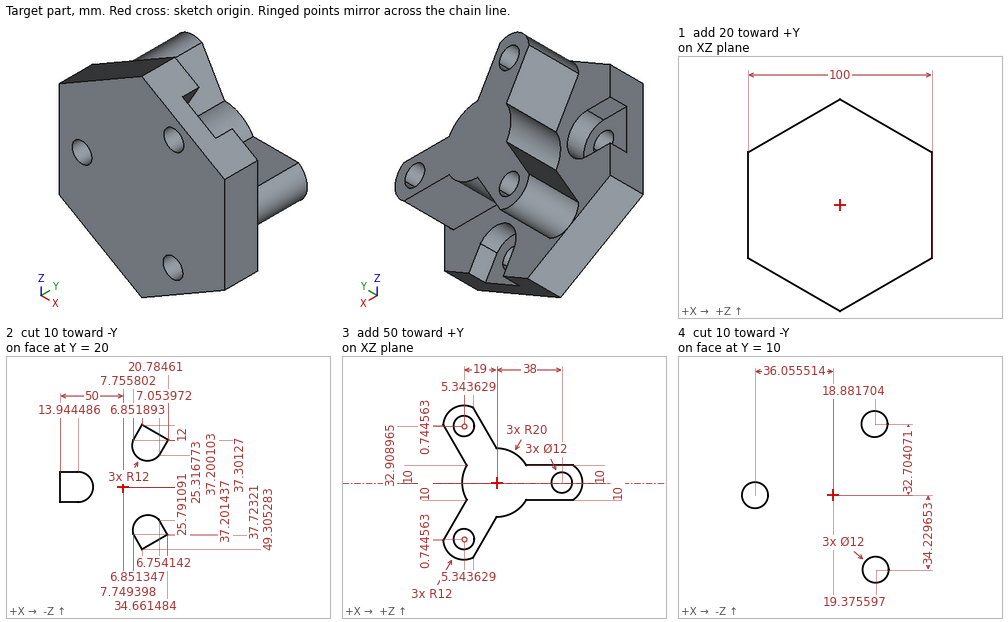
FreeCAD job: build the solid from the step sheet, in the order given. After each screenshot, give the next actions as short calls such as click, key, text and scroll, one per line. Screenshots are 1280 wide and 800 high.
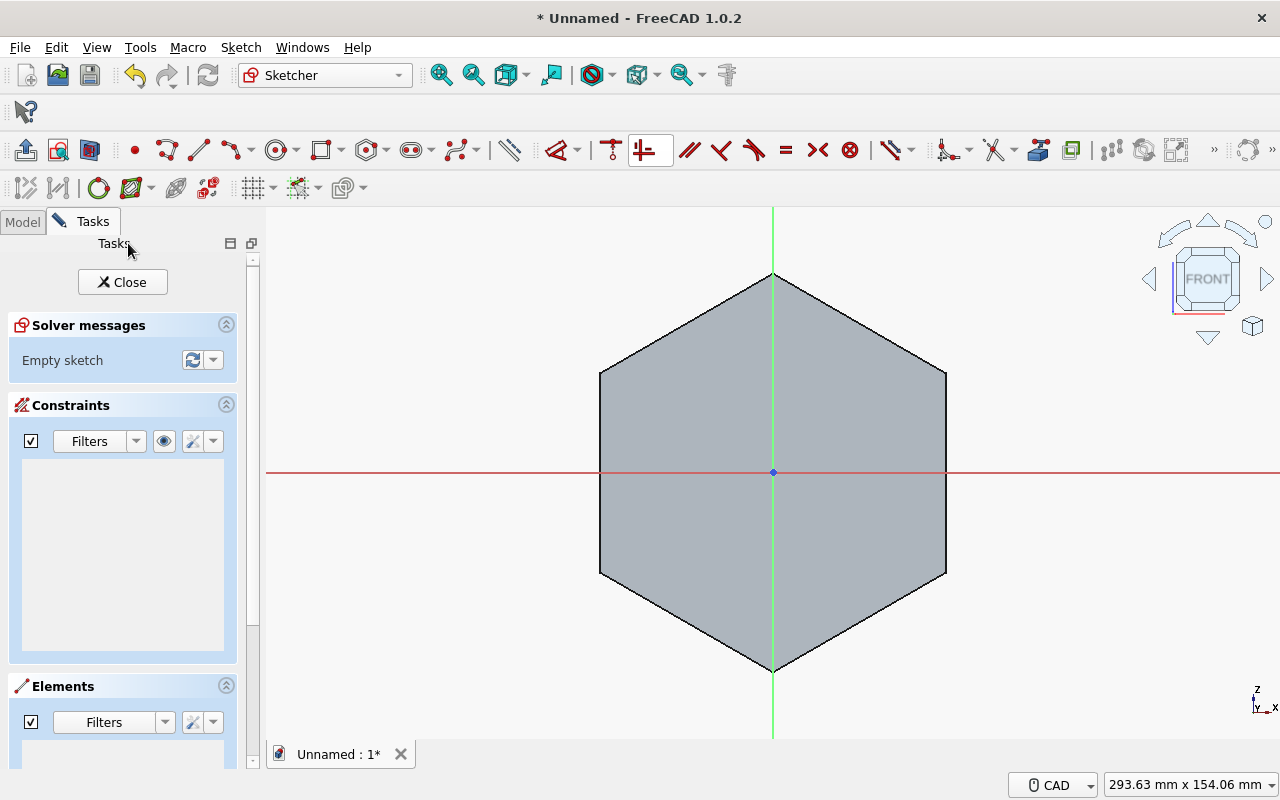
click(200, 150)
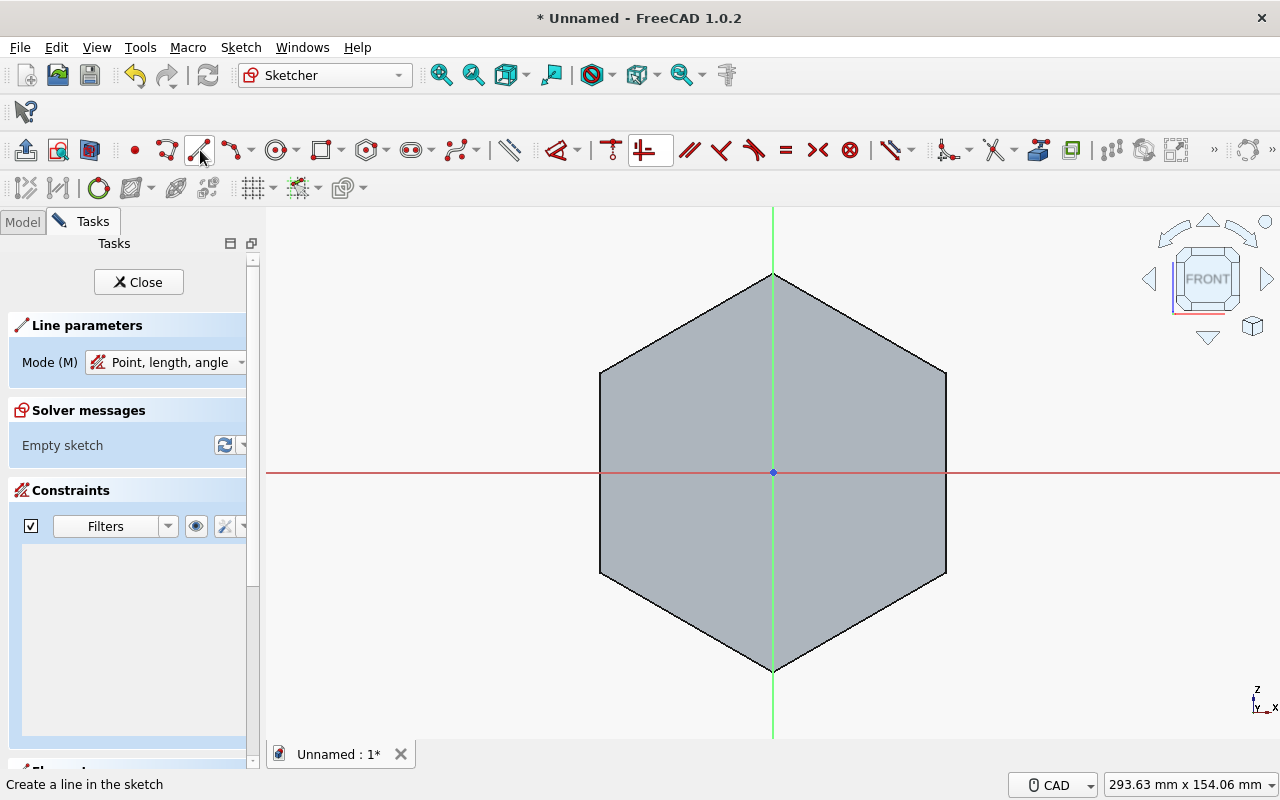
click(833, 438)
click(927, 438)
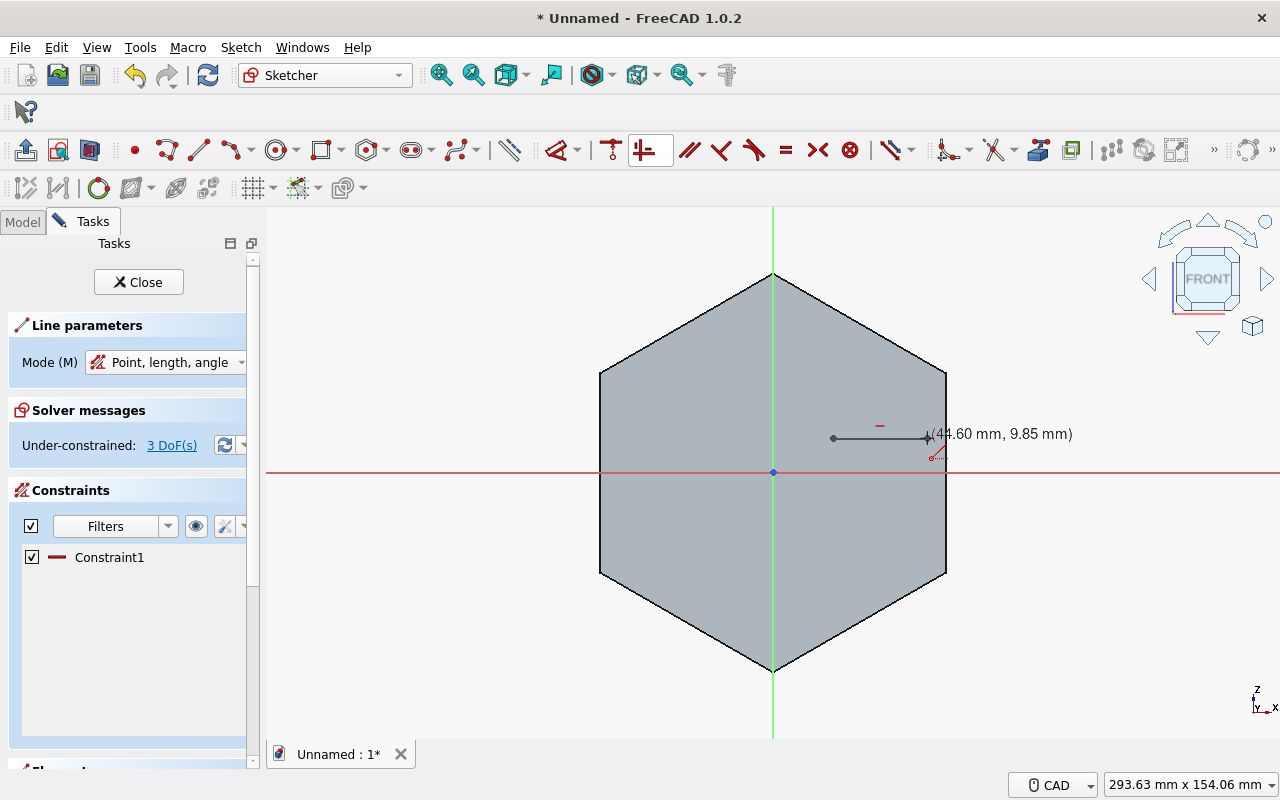
click(927, 508)
click(833, 508)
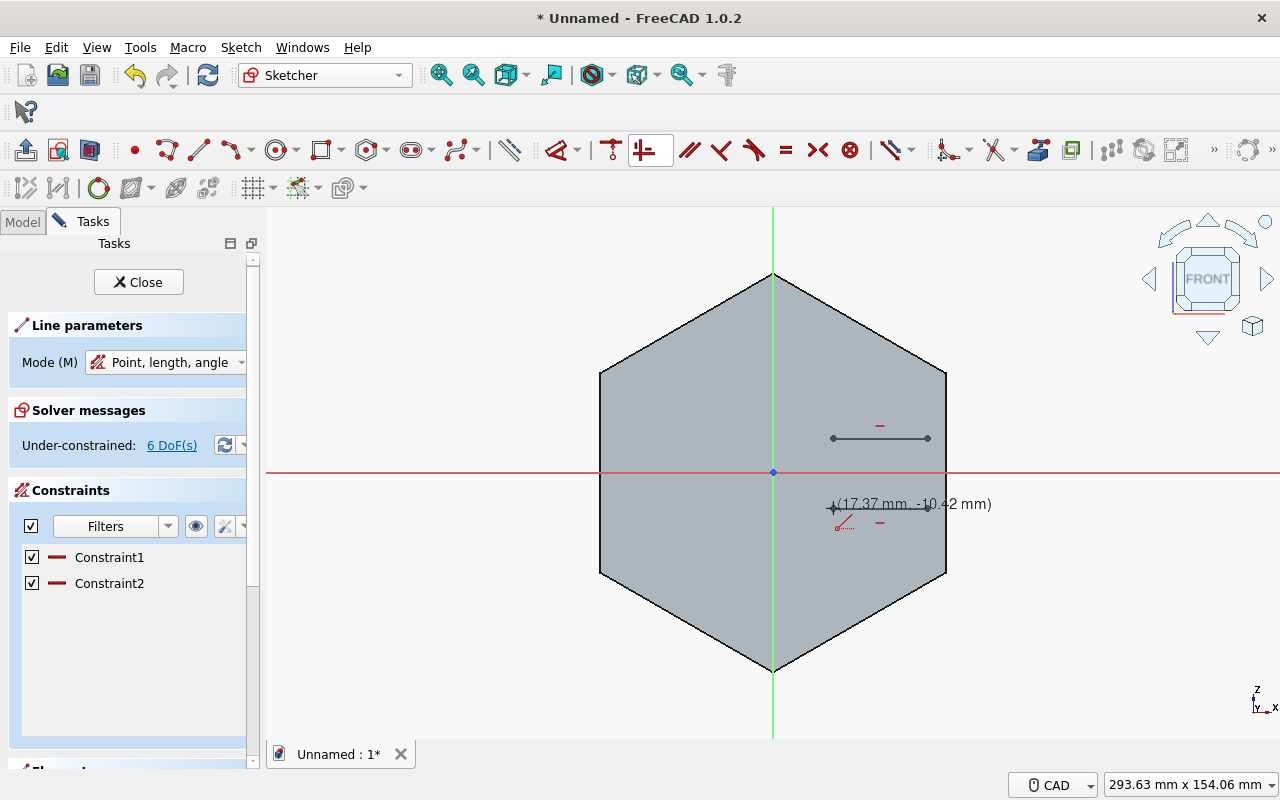
click(773, 542)
click(726, 624)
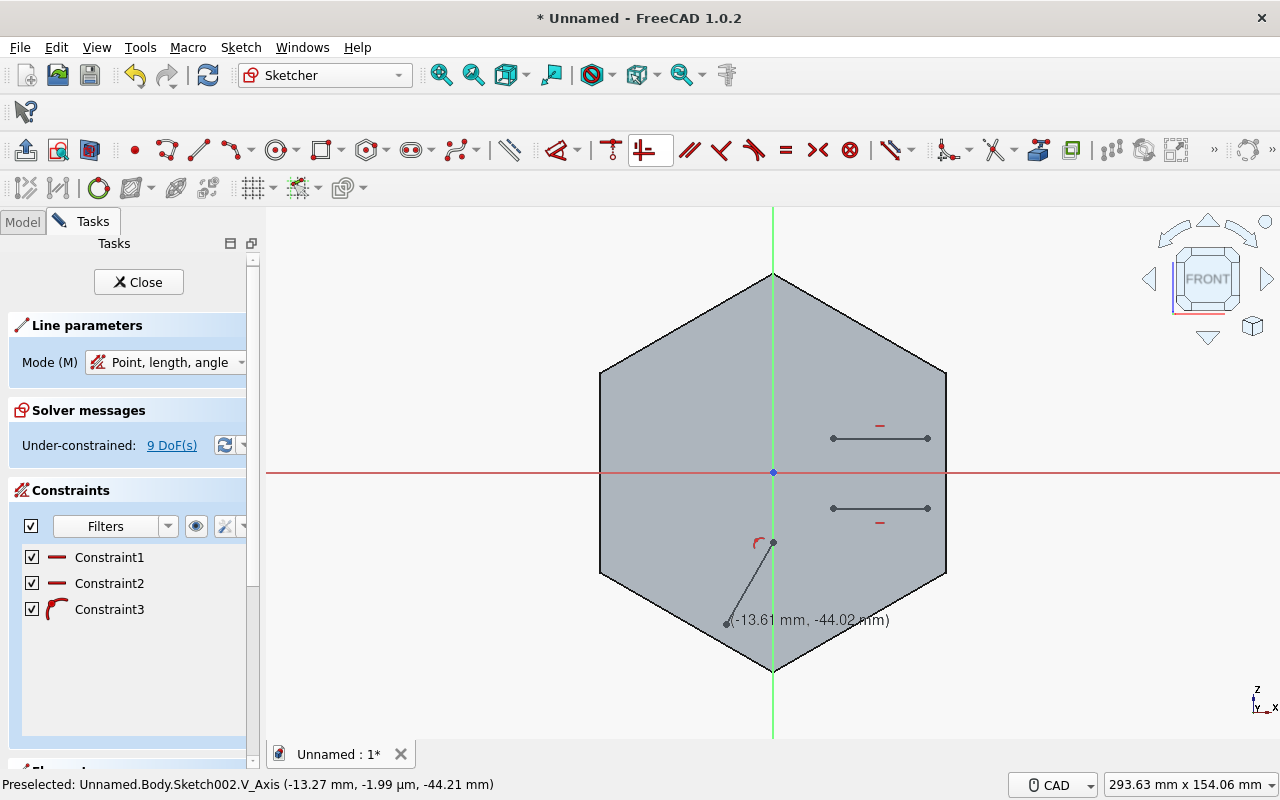
click(666, 589)
click(713, 508)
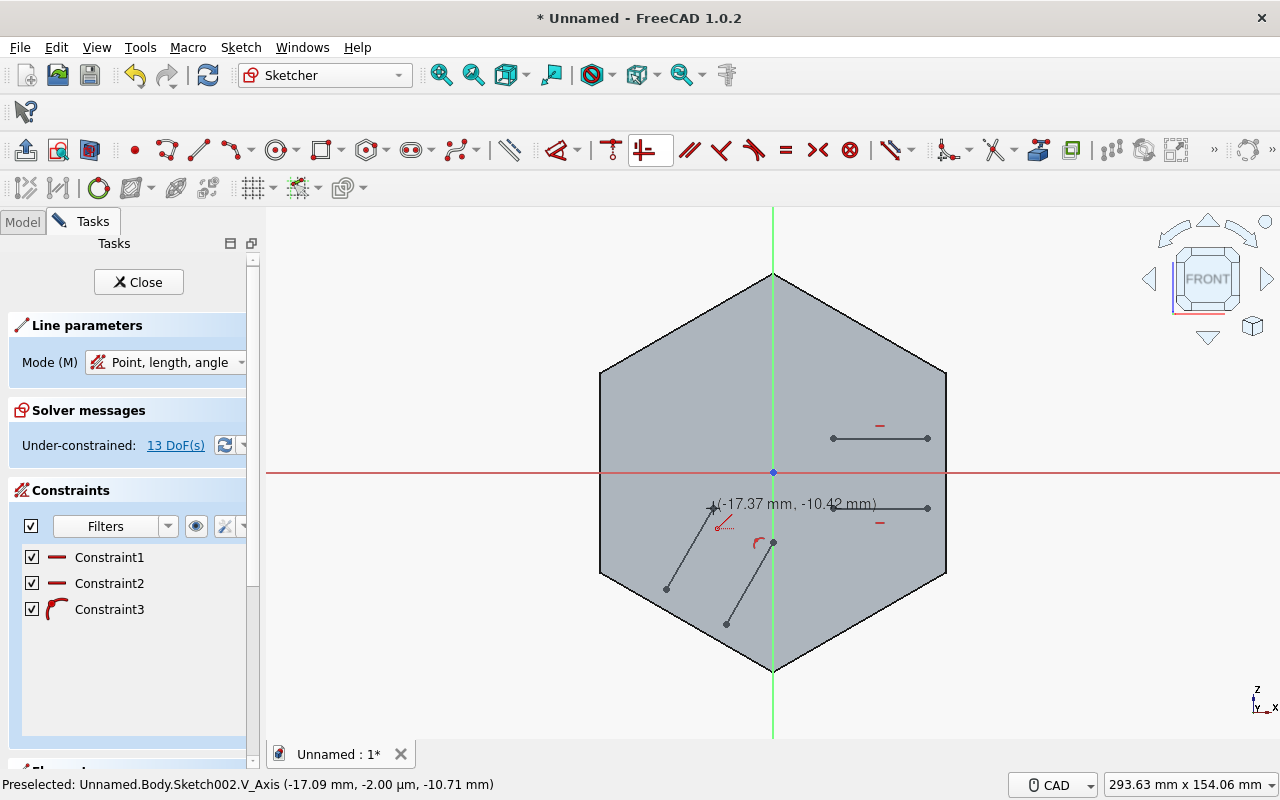
click(713, 438)
click(666, 357)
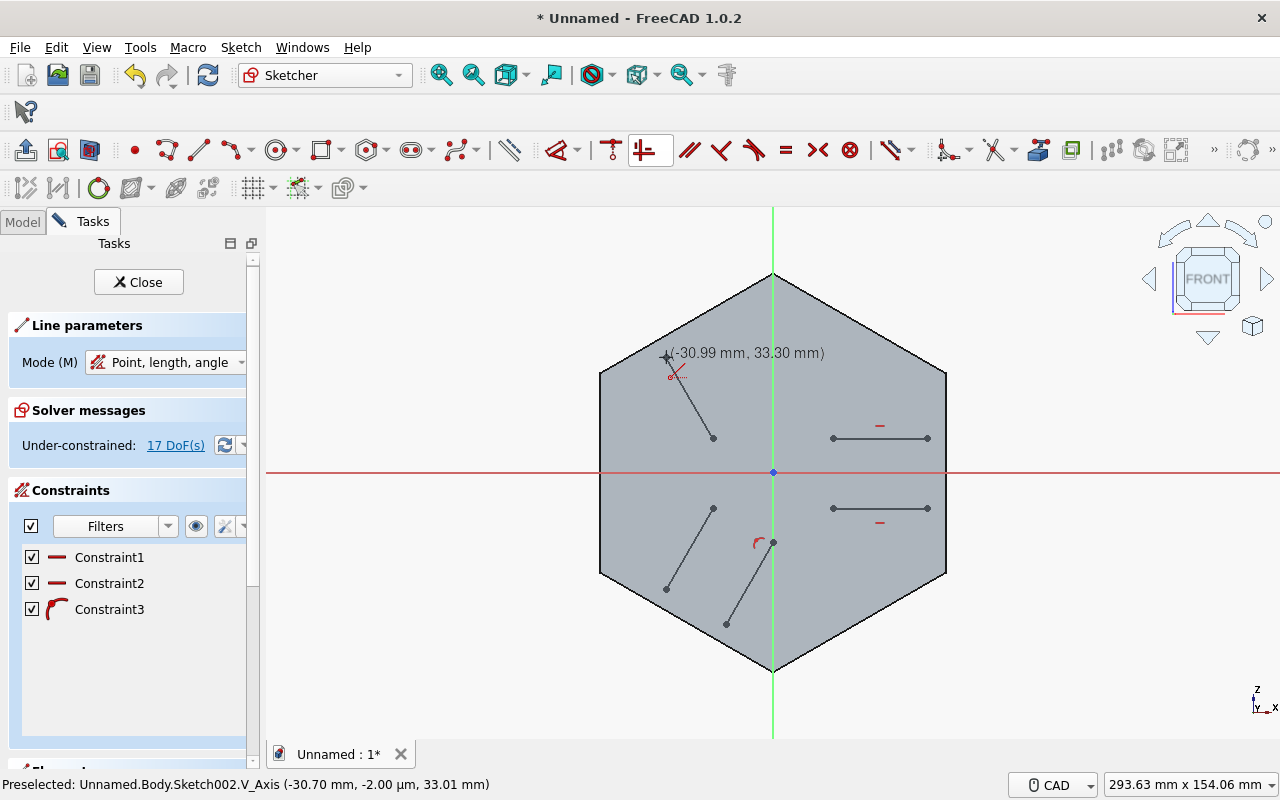
click(726, 322)
click(773, 404)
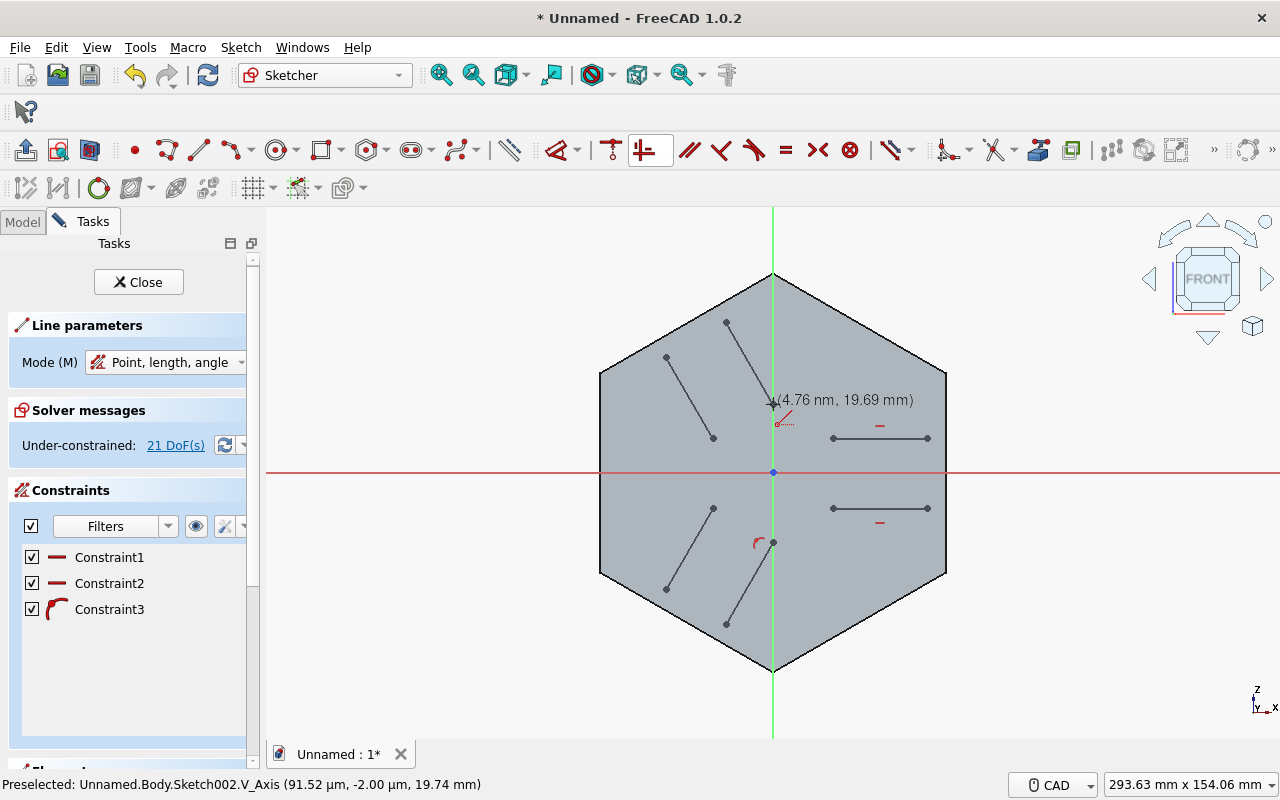
click(232, 150)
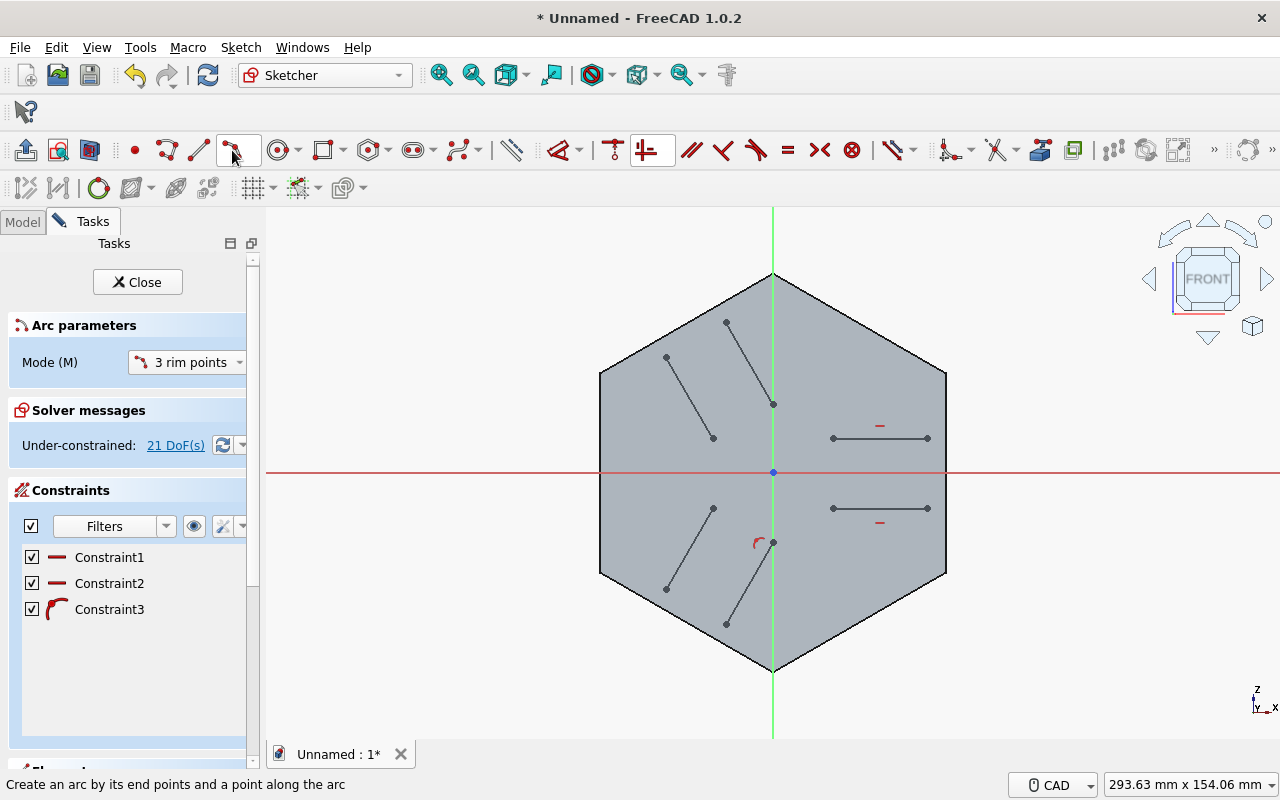
click(927, 439)
click(927, 509)
click(942, 489)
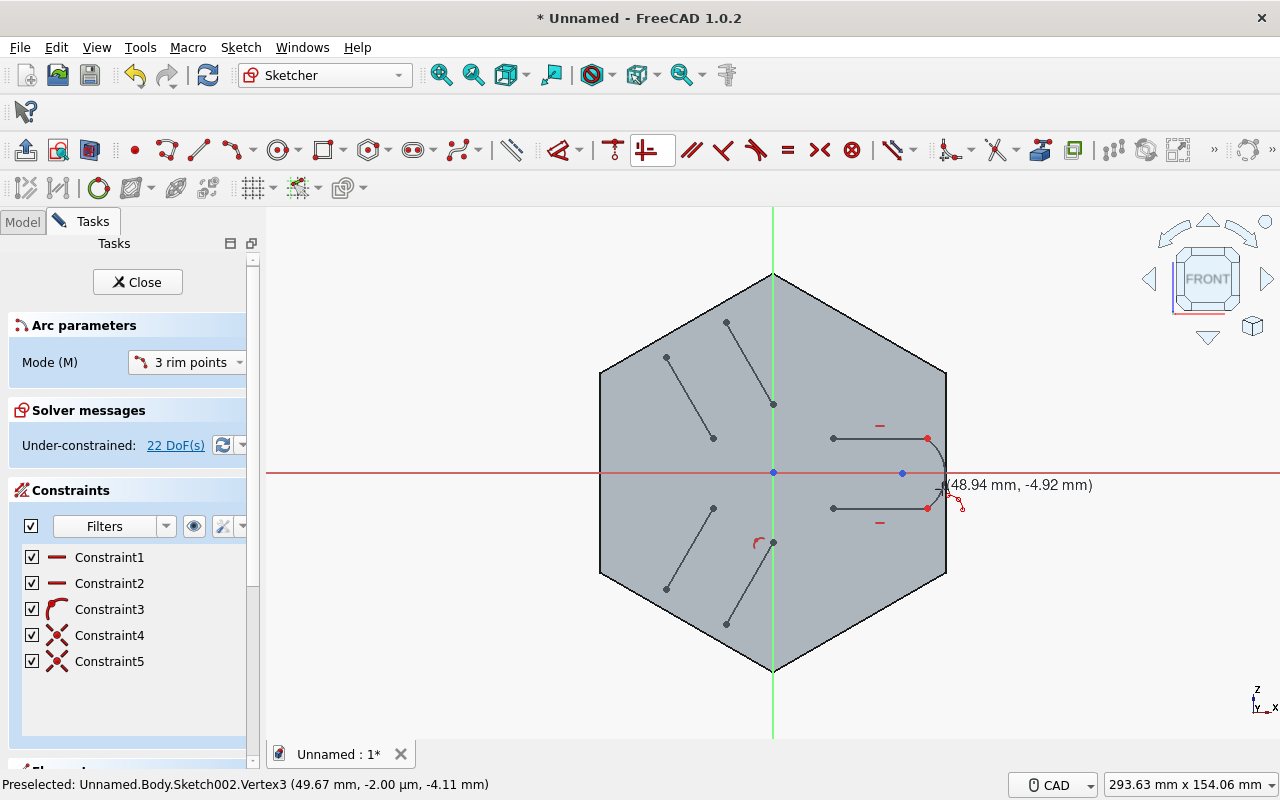
click(833, 509)
click(773, 543)